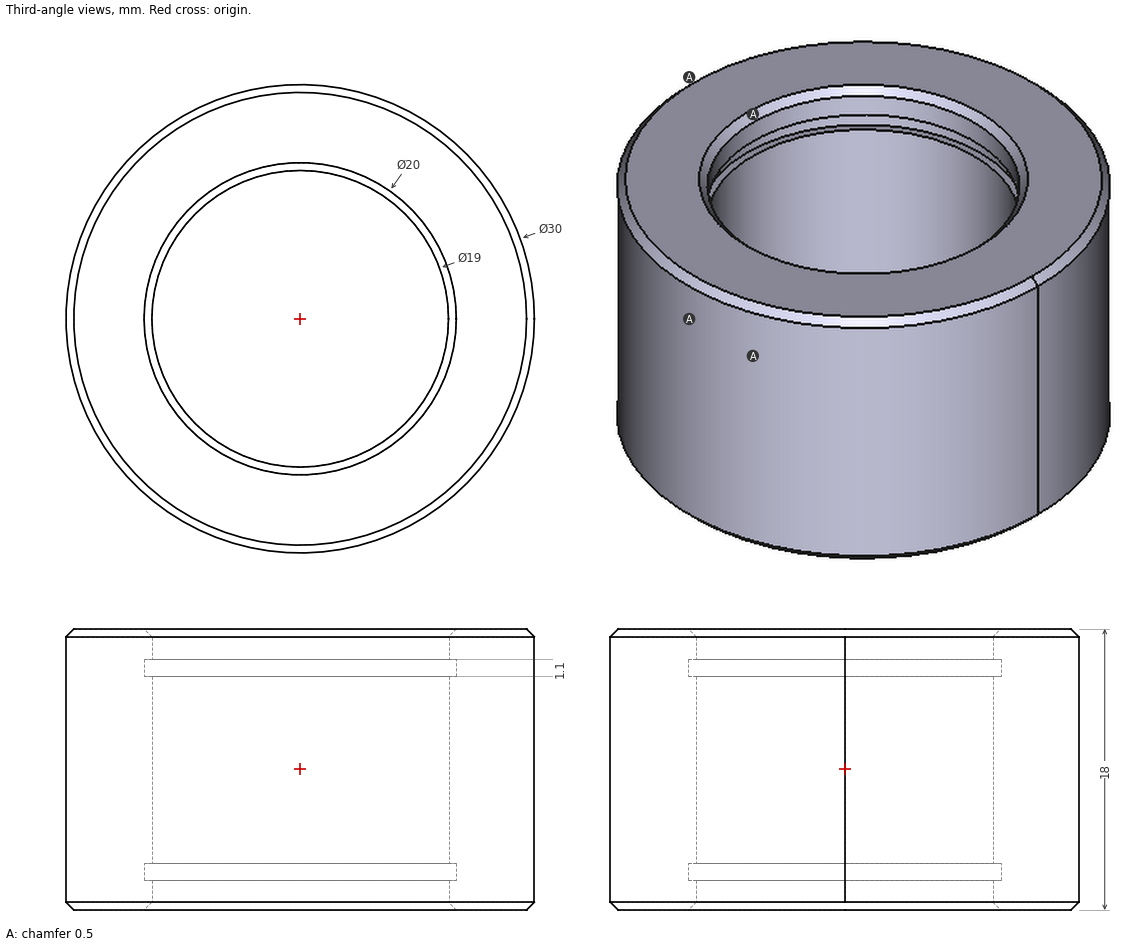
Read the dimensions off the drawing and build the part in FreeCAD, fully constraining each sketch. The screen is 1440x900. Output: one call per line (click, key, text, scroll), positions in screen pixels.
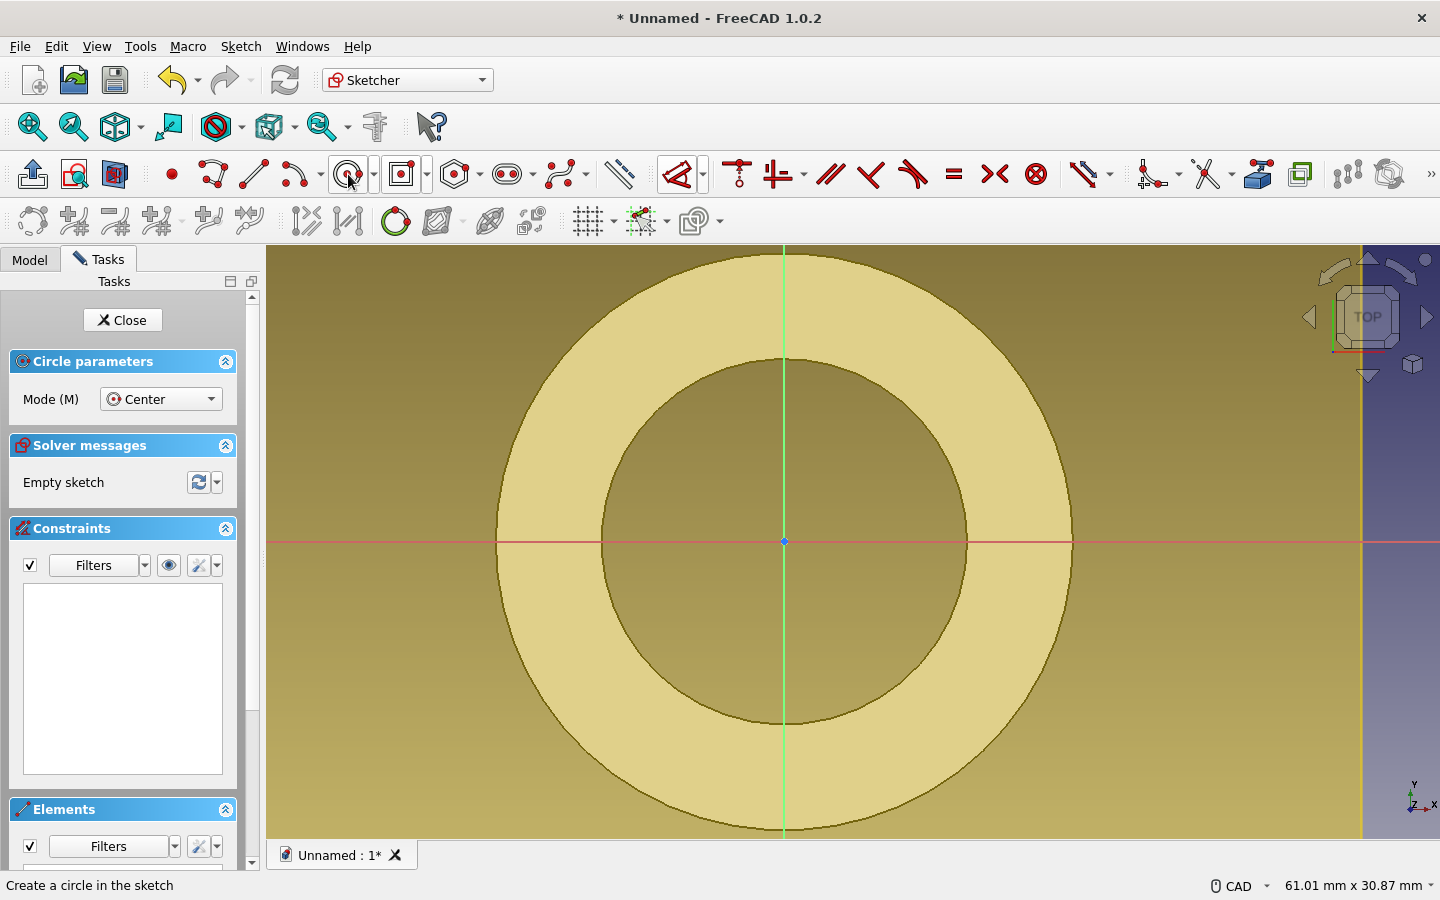
click(784, 542)
click(920, 406)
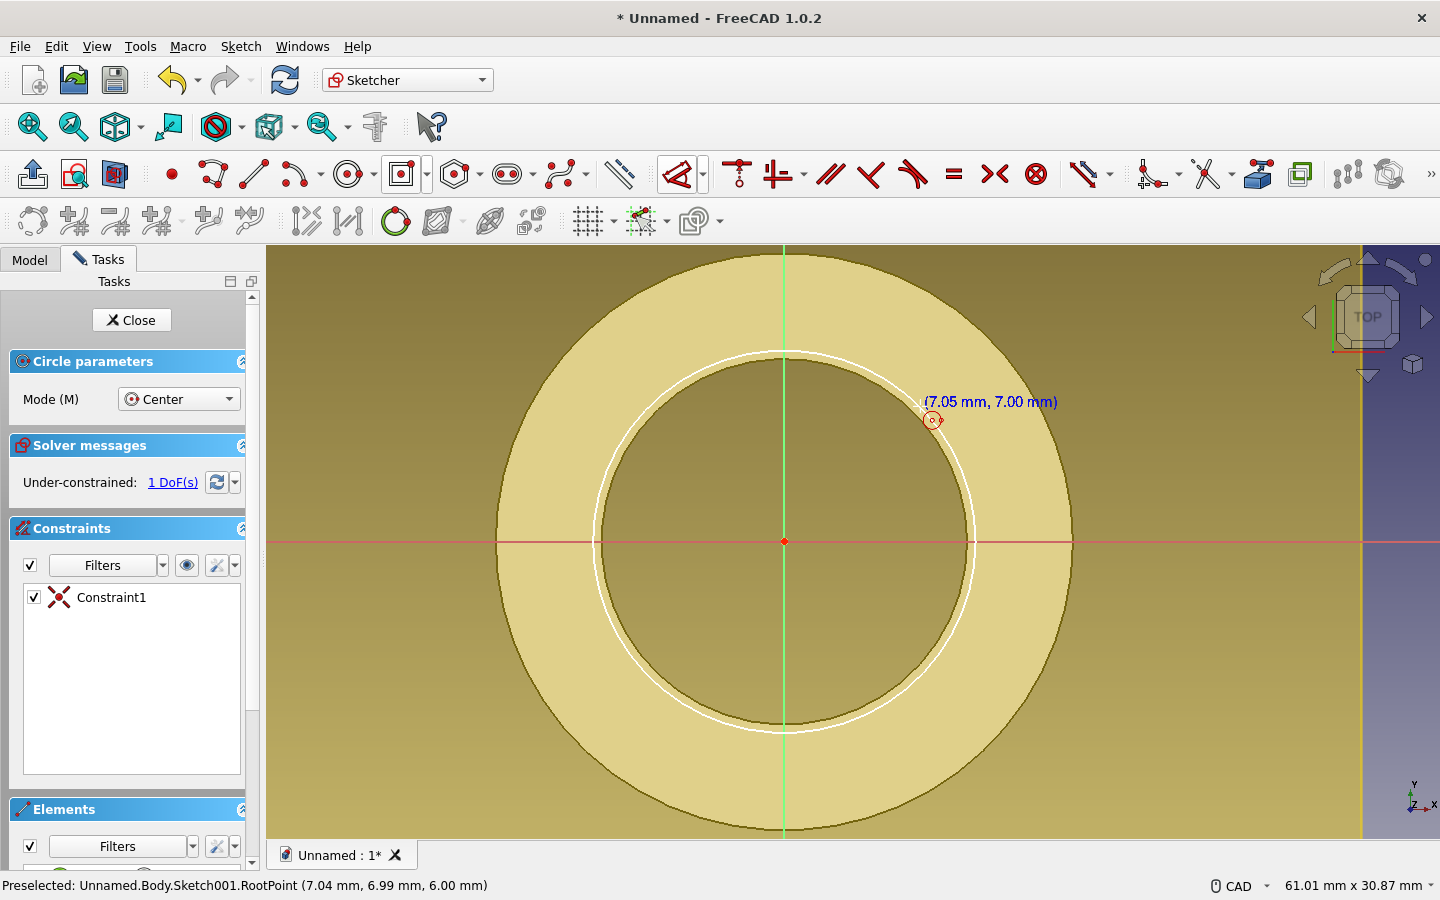
click(784, 542)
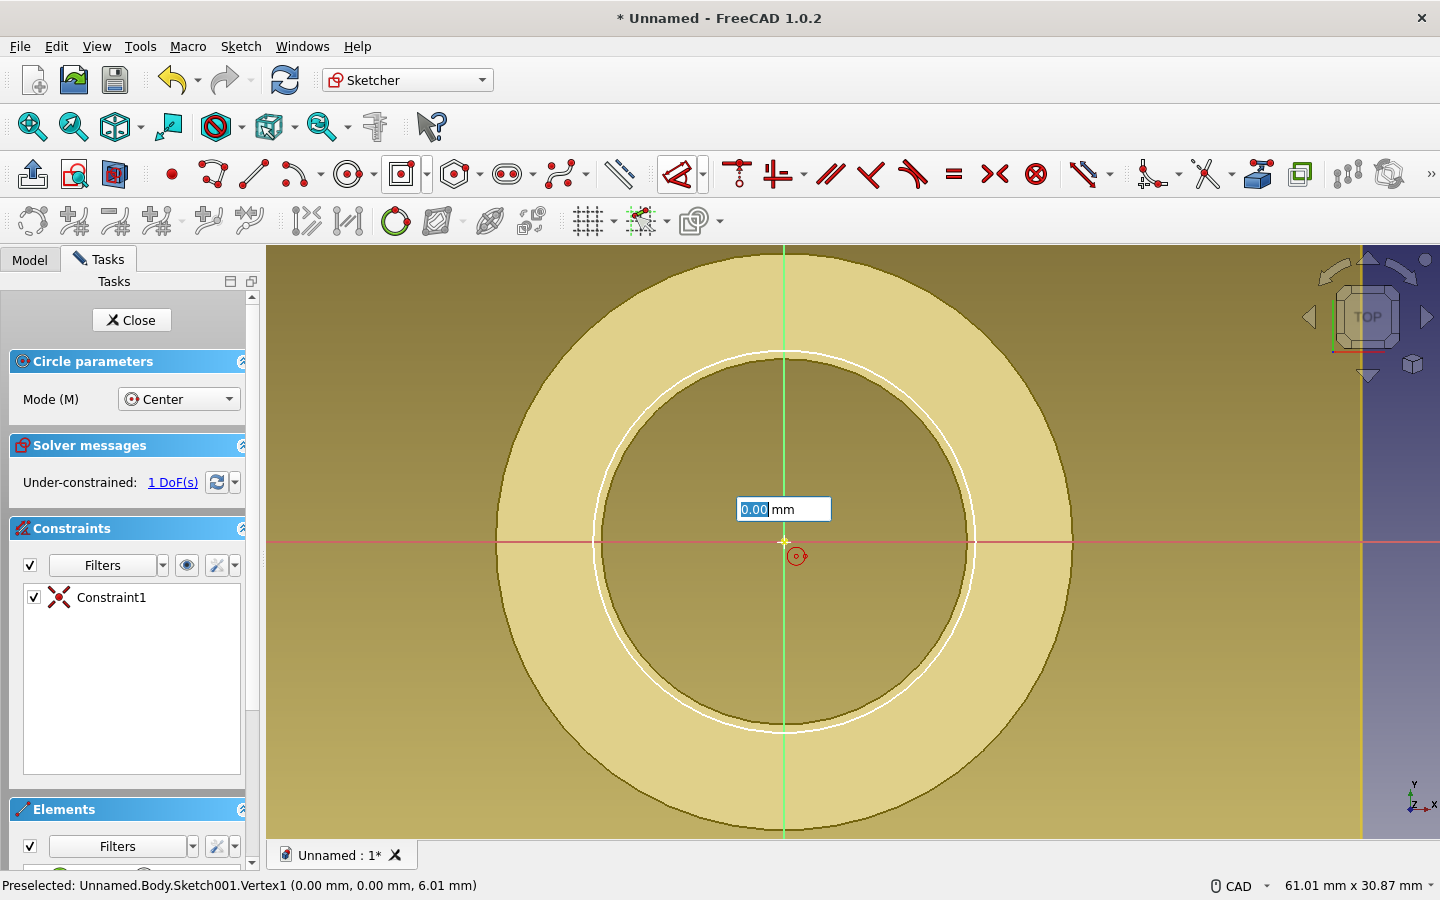
scroll(914, 412, up, 3)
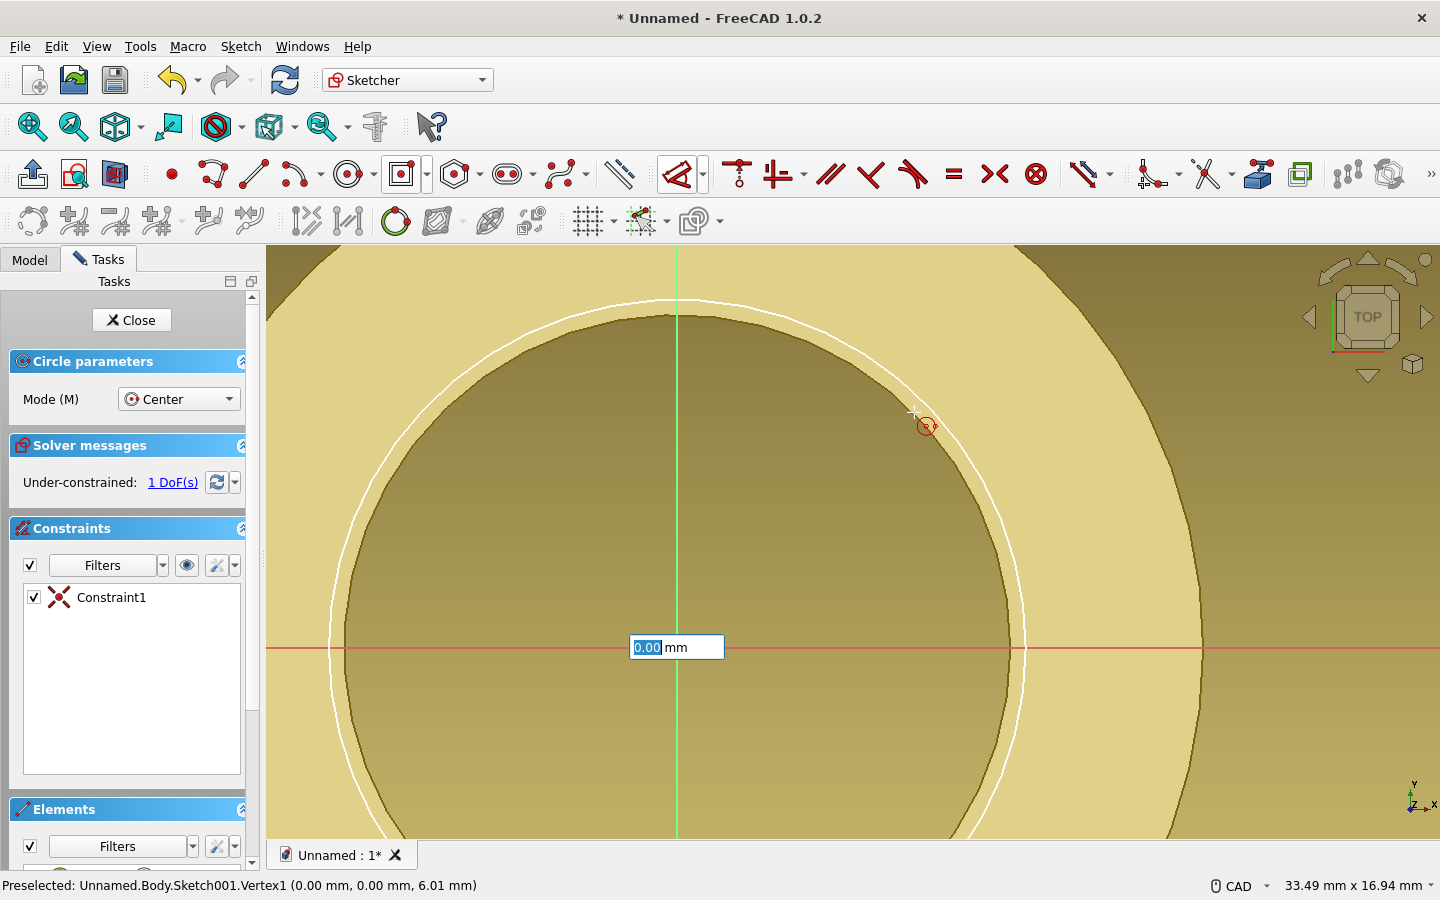
click(913, 413)
key(Escape)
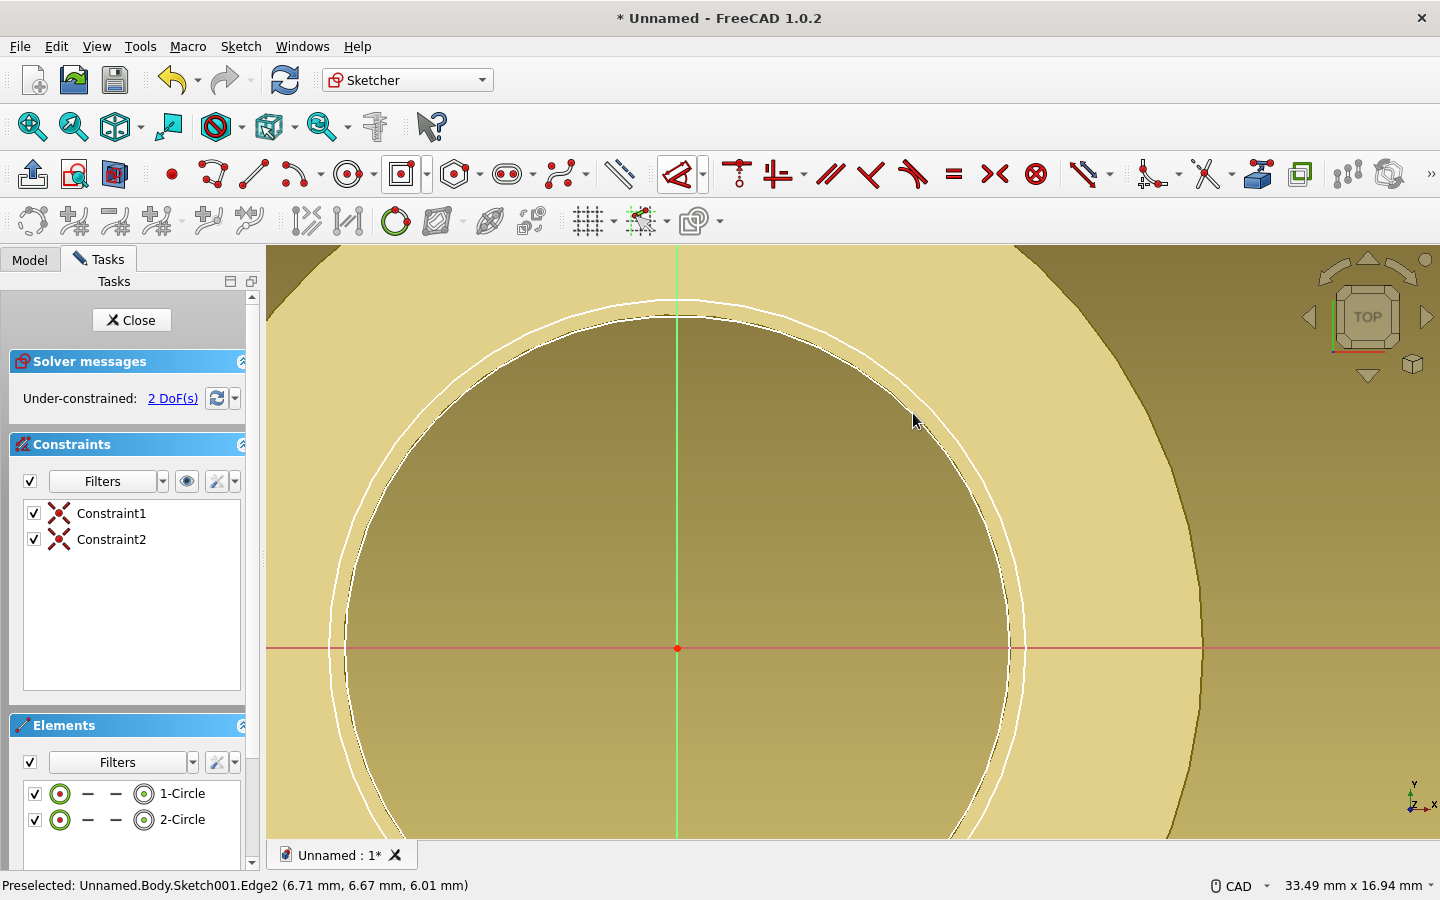
click(923, 401)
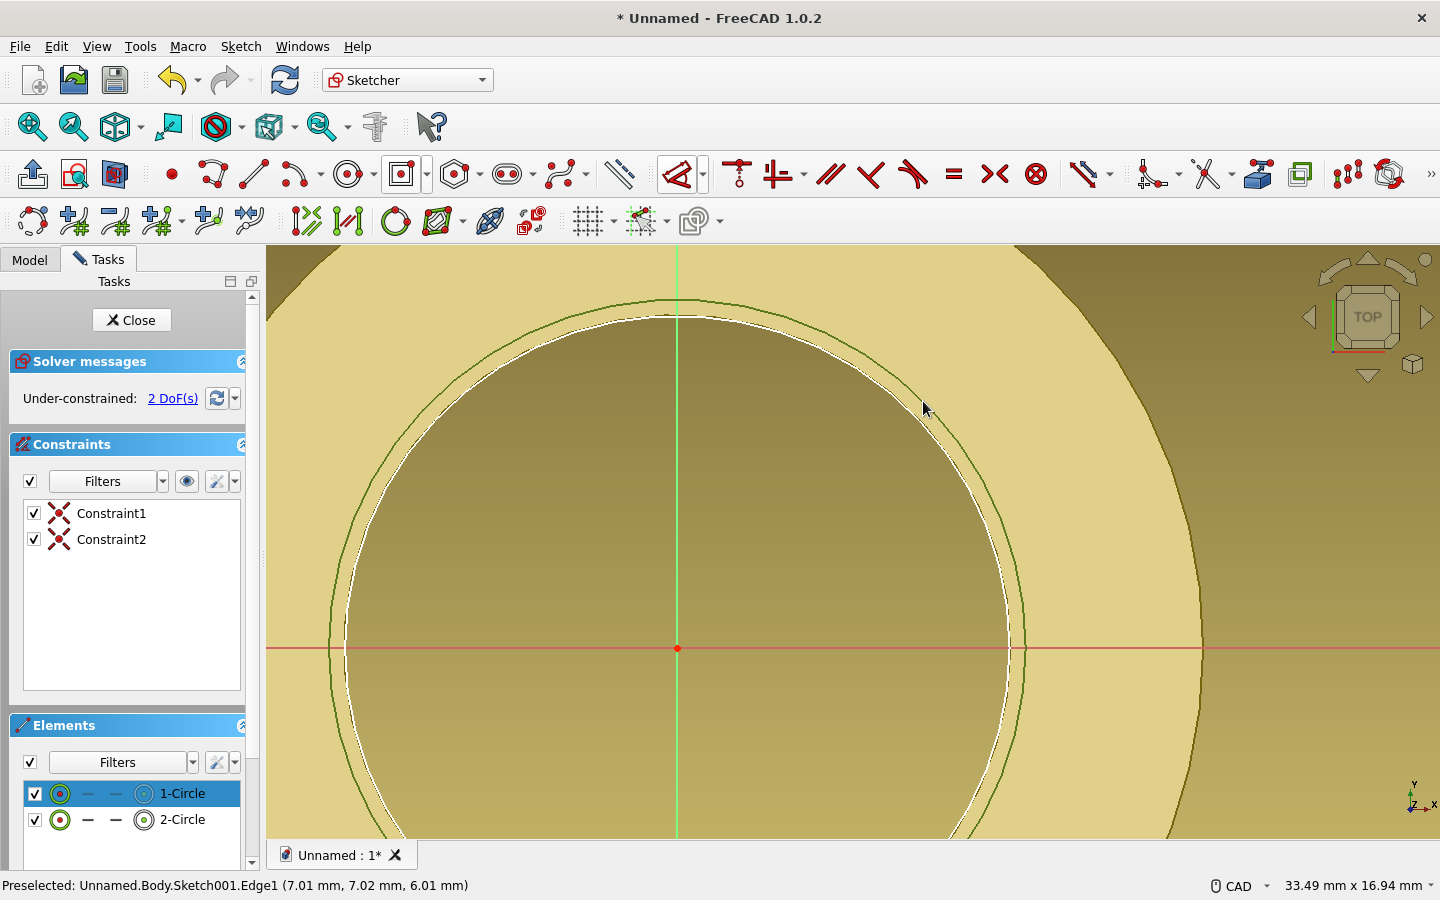
key(k)
key(o)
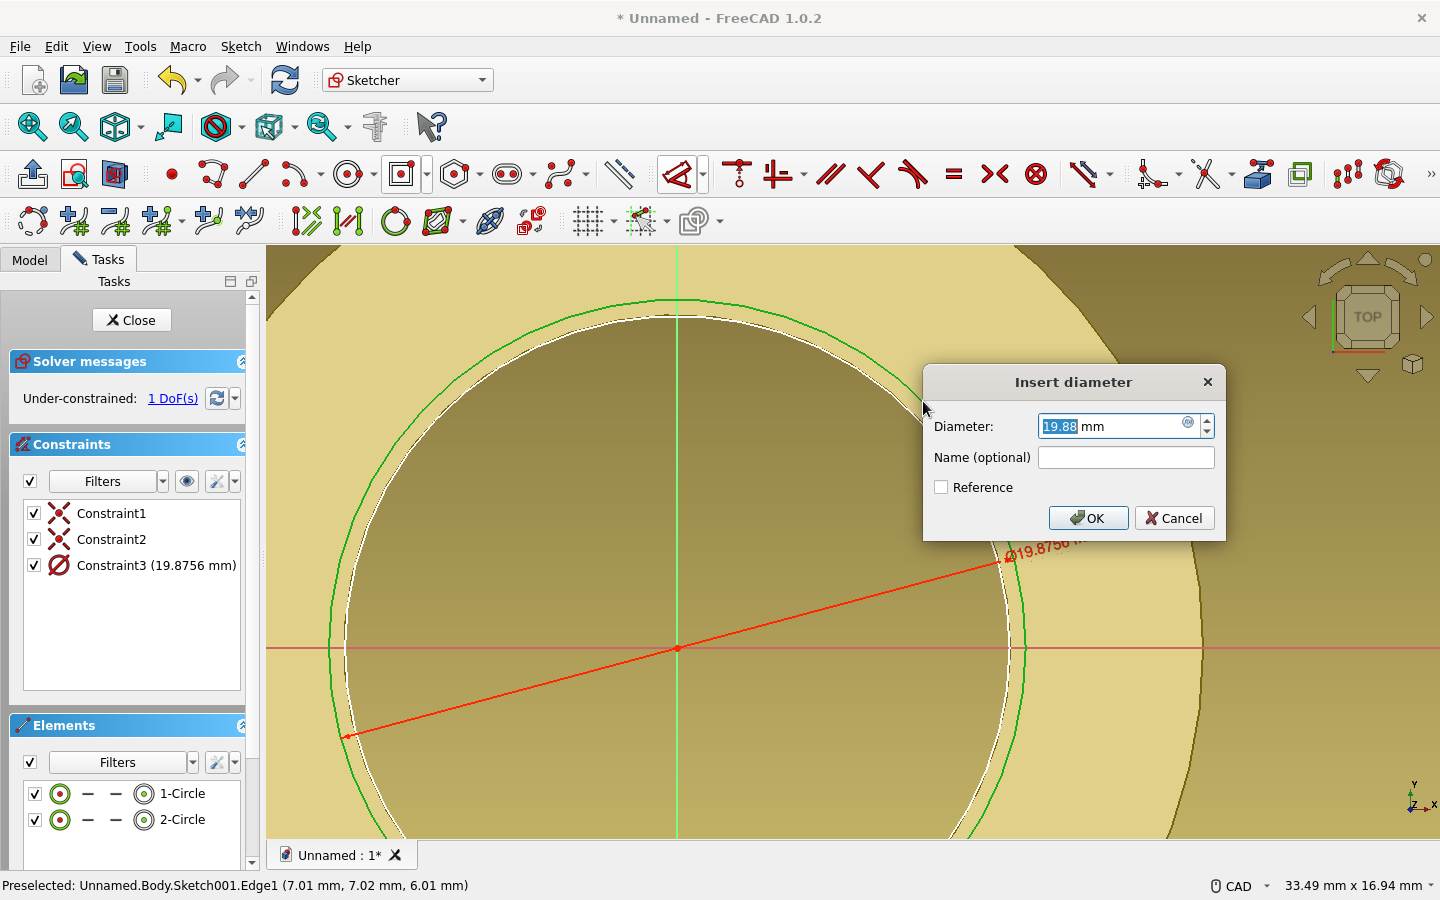
text(20)
key(Return)